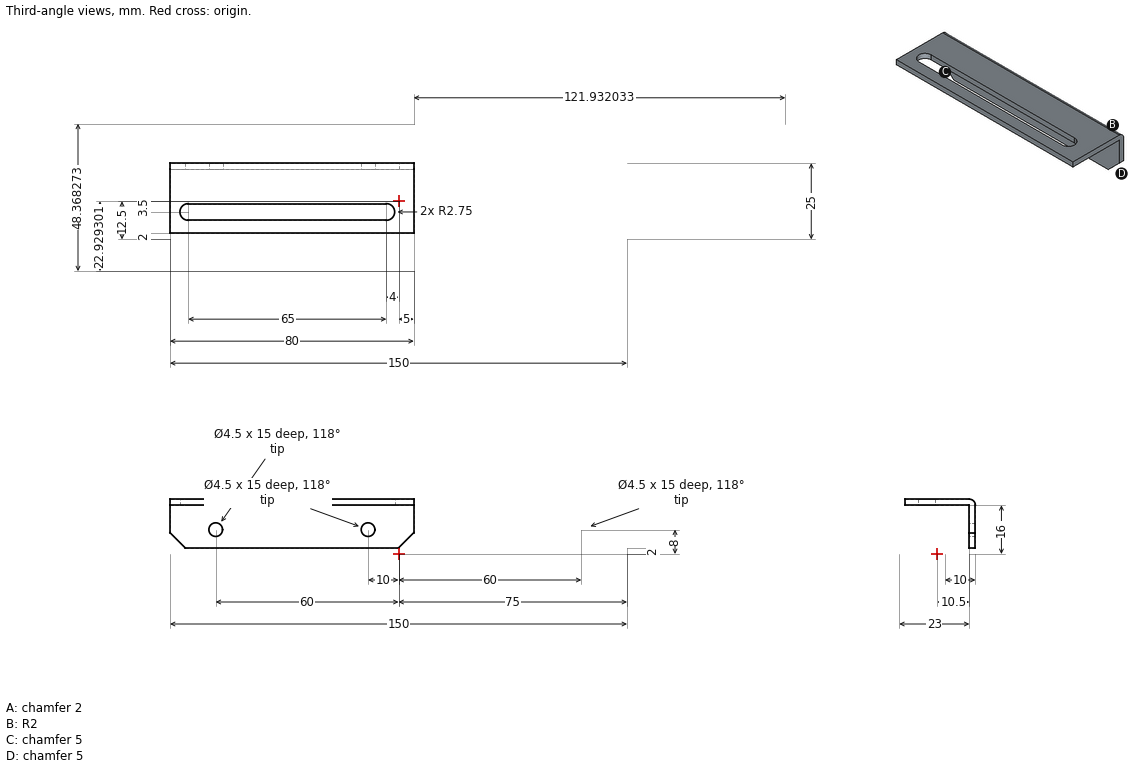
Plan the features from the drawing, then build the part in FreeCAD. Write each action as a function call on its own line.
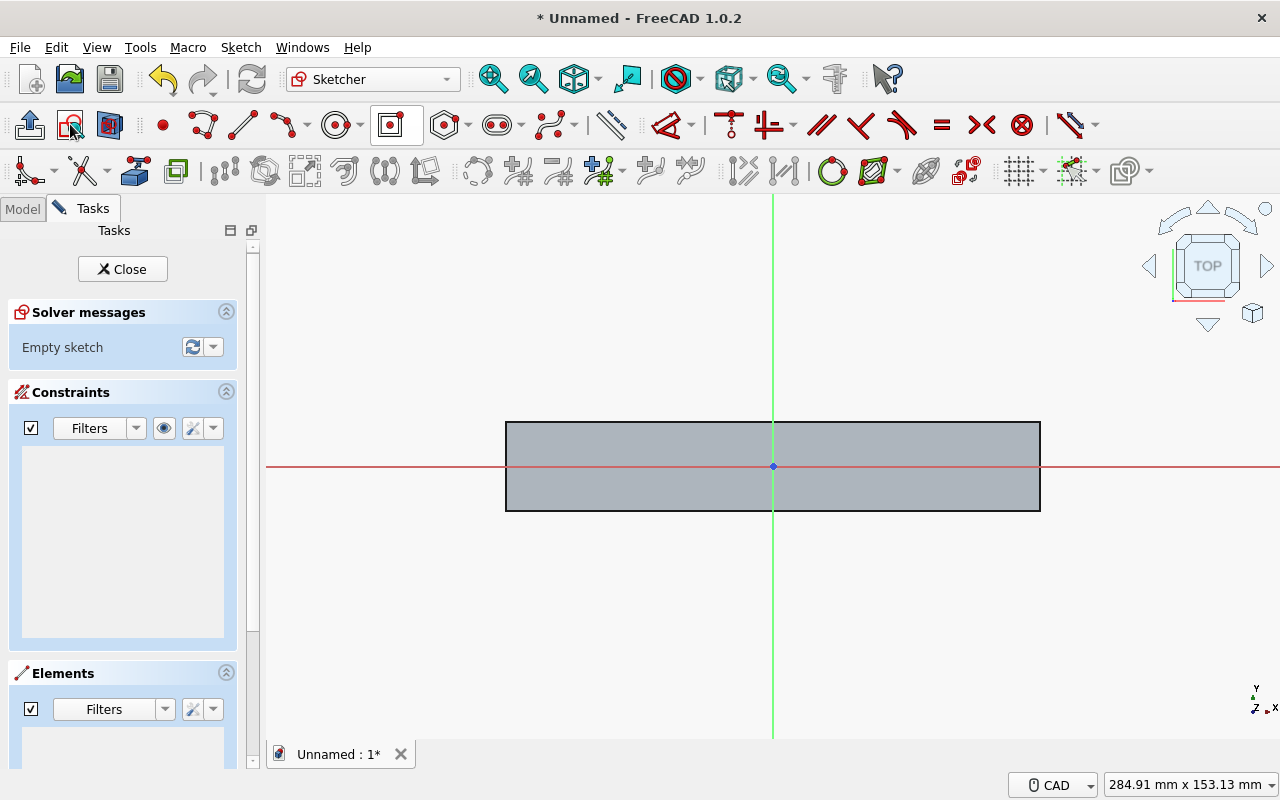
scroll(597, 487, up, 4)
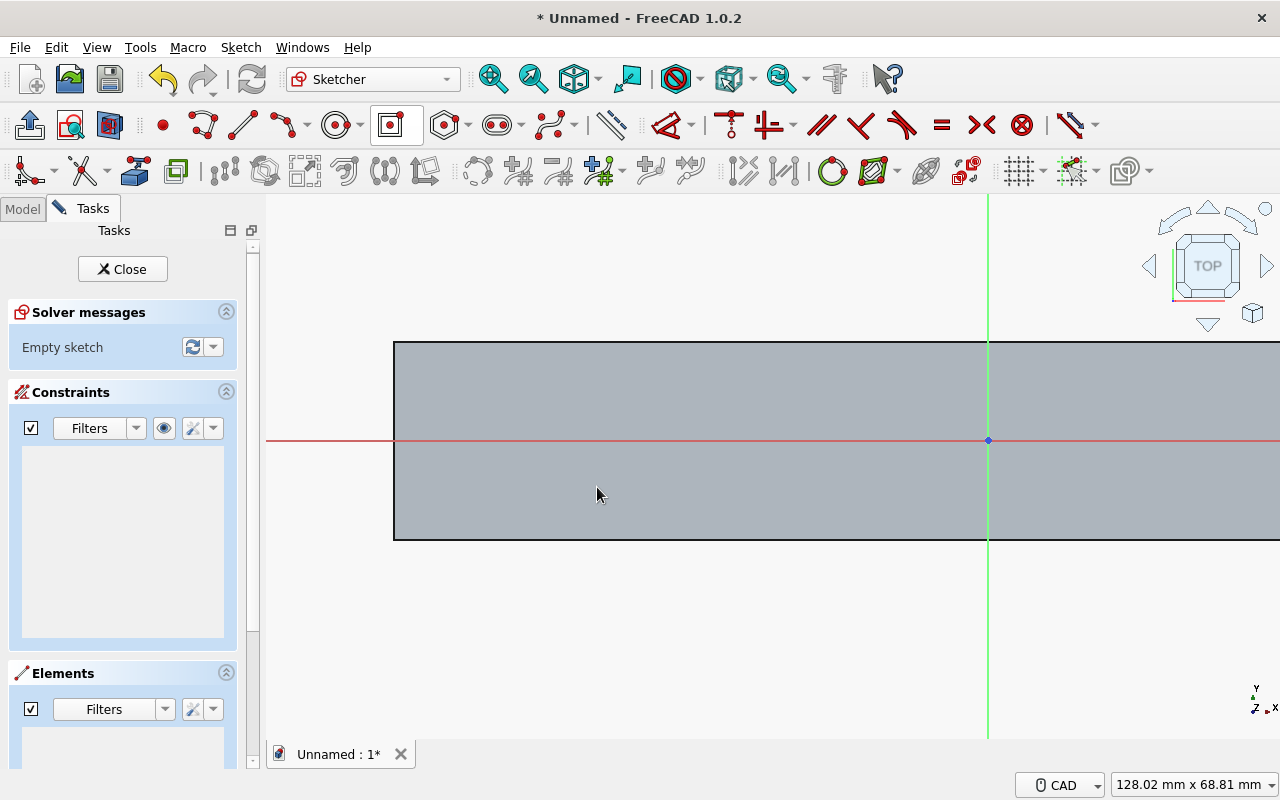
click(498, 126)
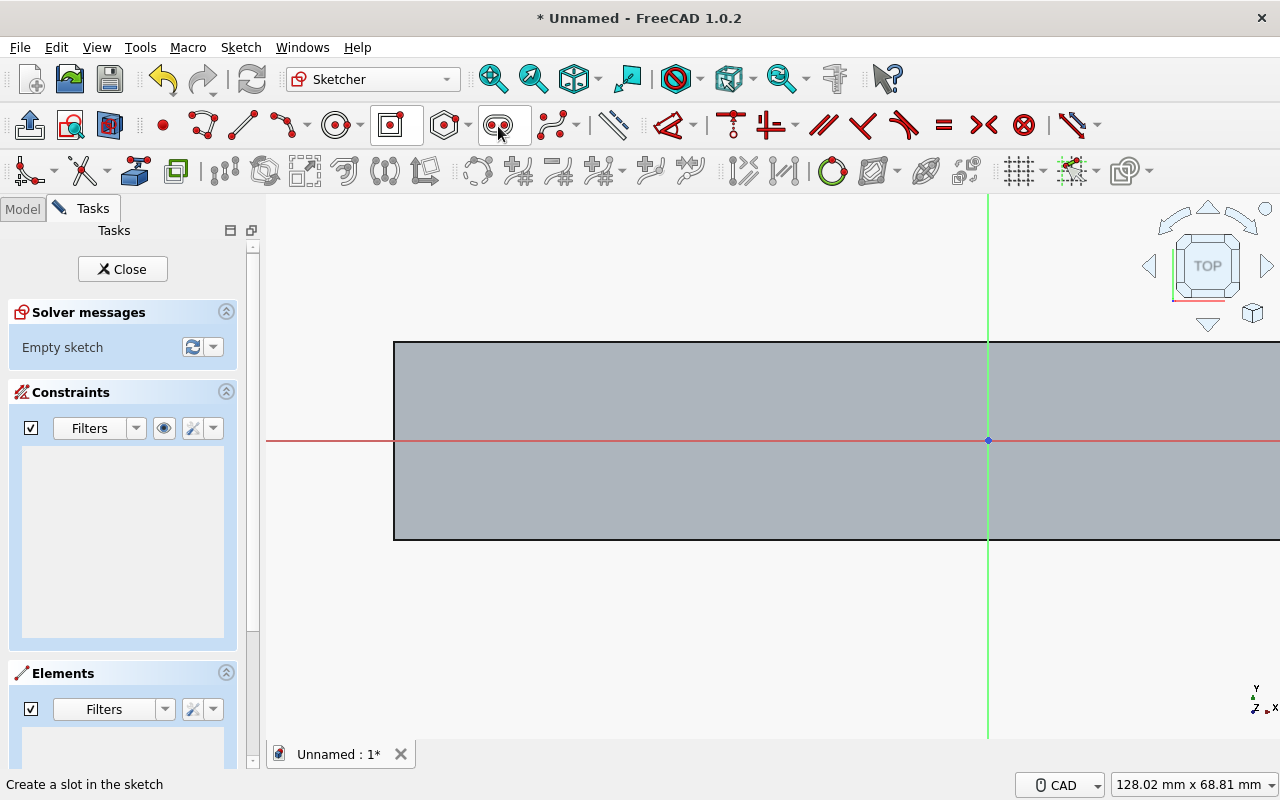
click(442, 468)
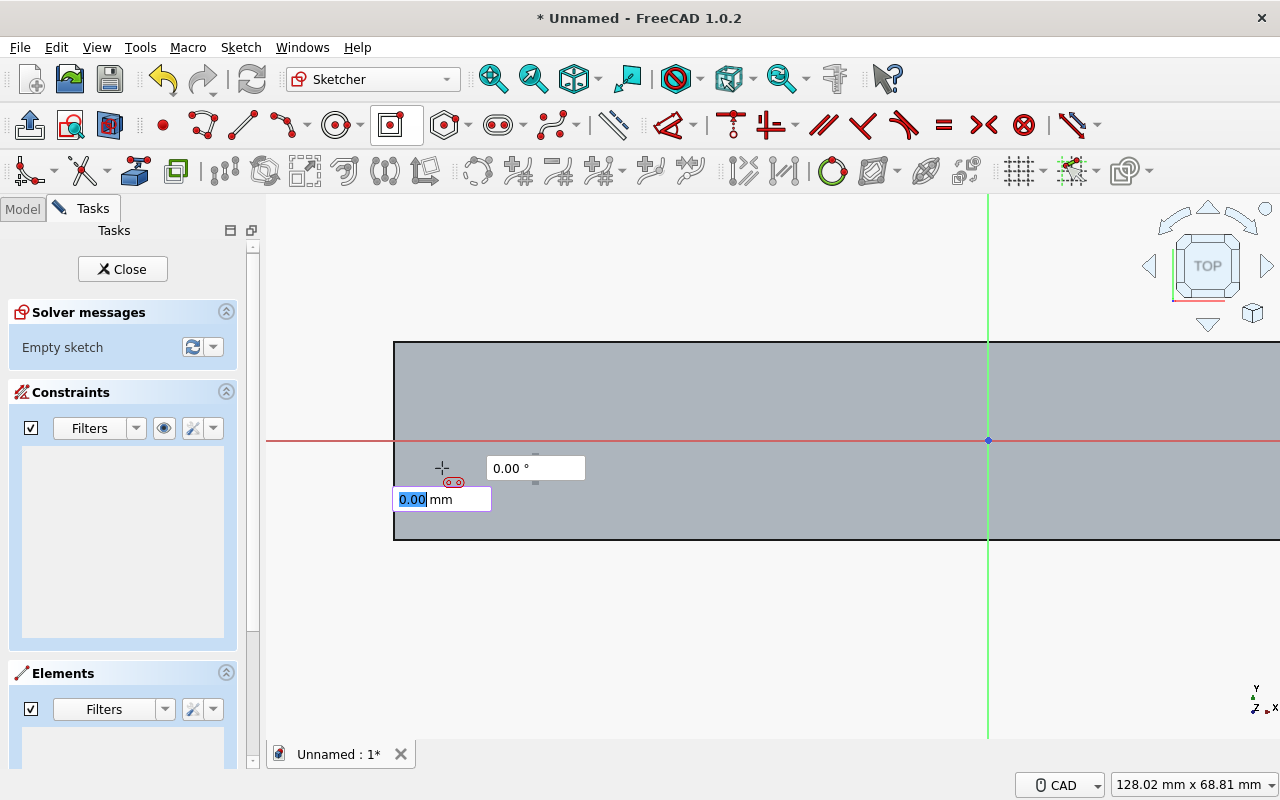
click(957, 468)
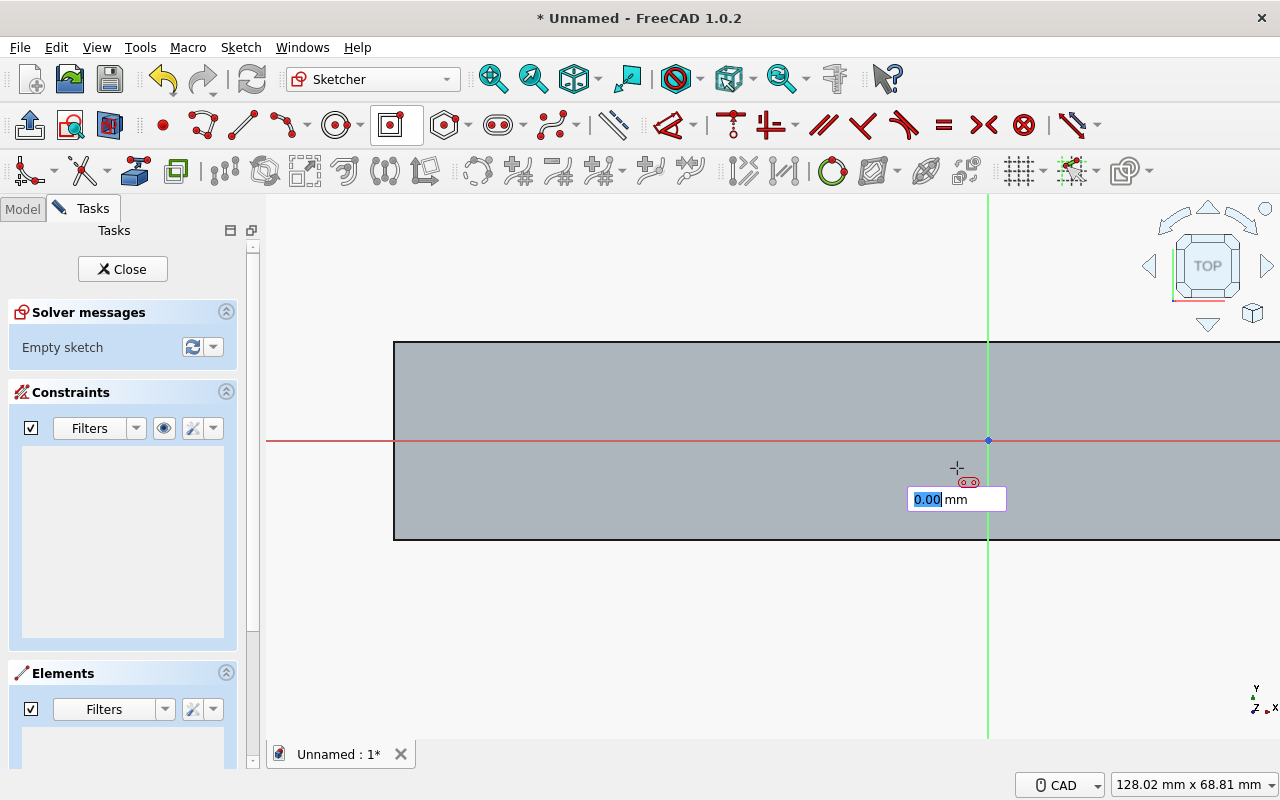
click(699, 490)
key(Escape)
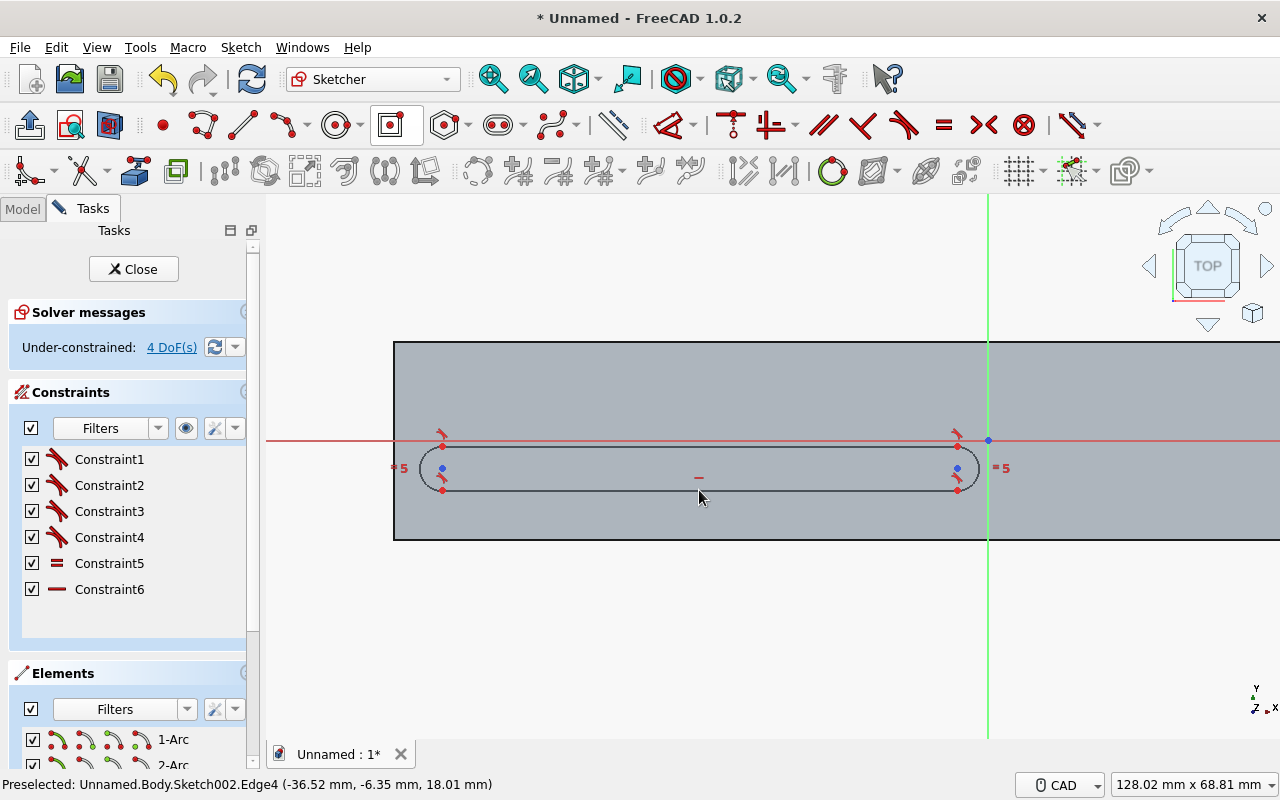
click(668, 126)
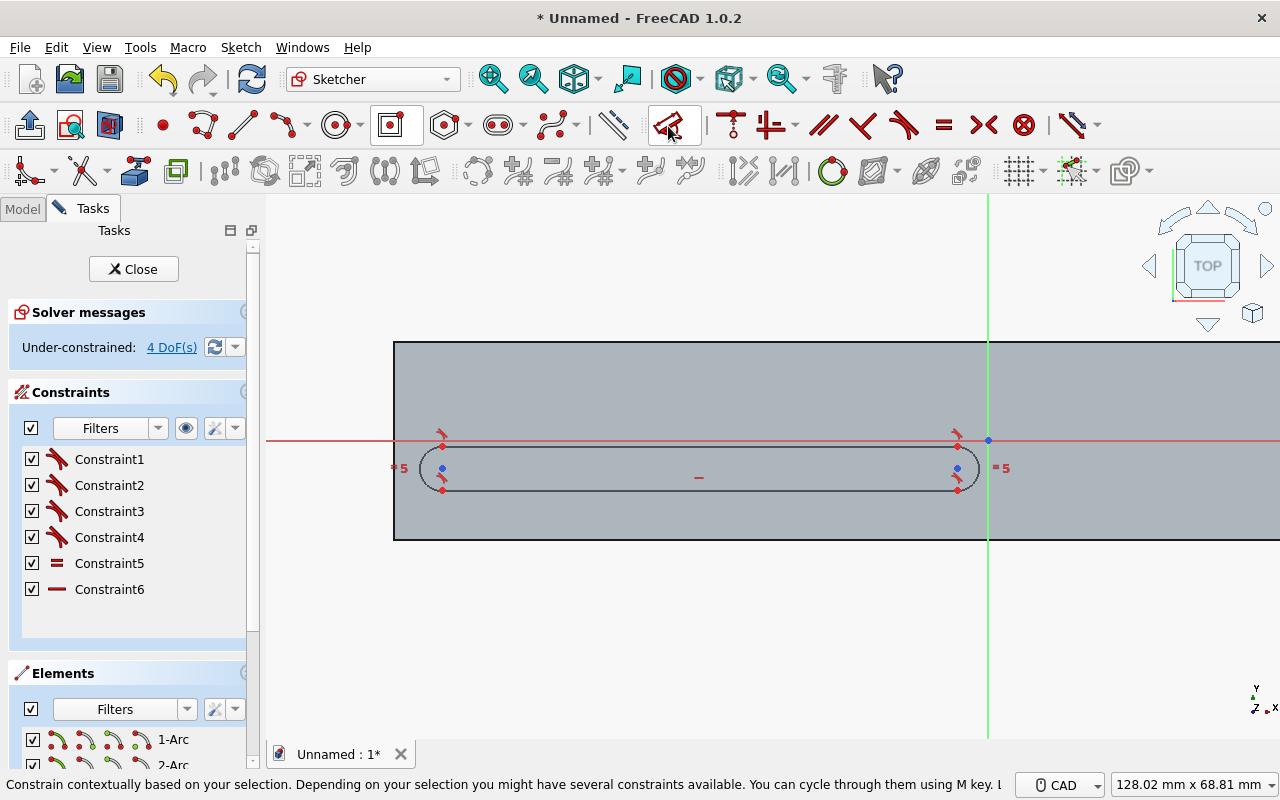
scroll(424, 456, up, 4)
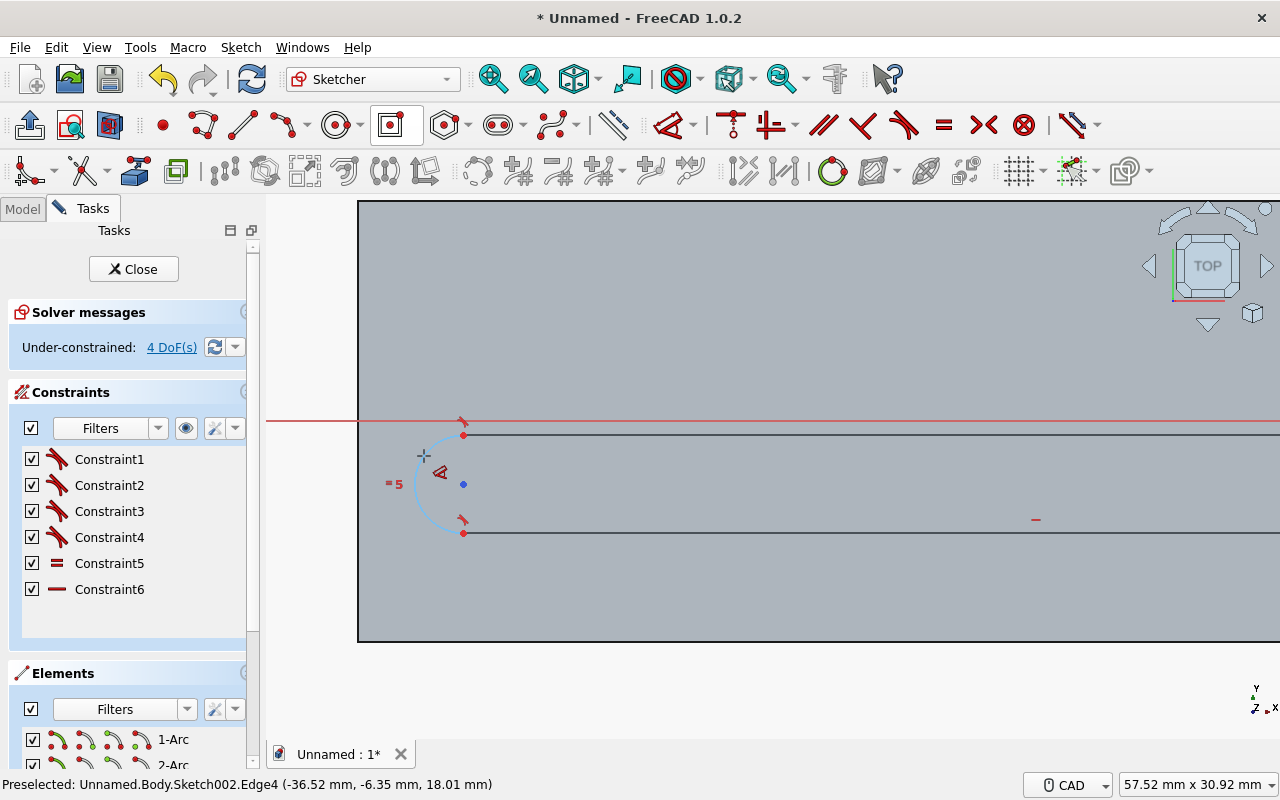
click(424, 456)
click(398, 437)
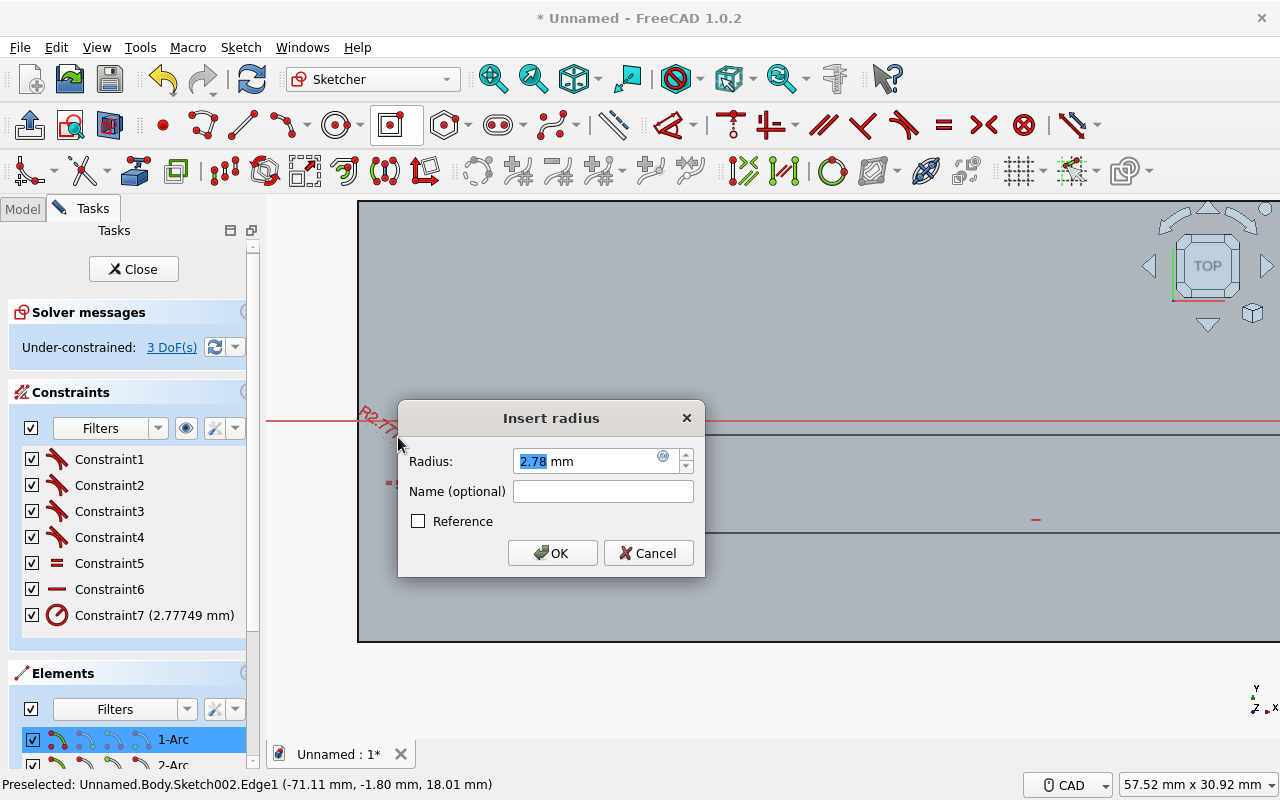
text(2.75)
key(Return)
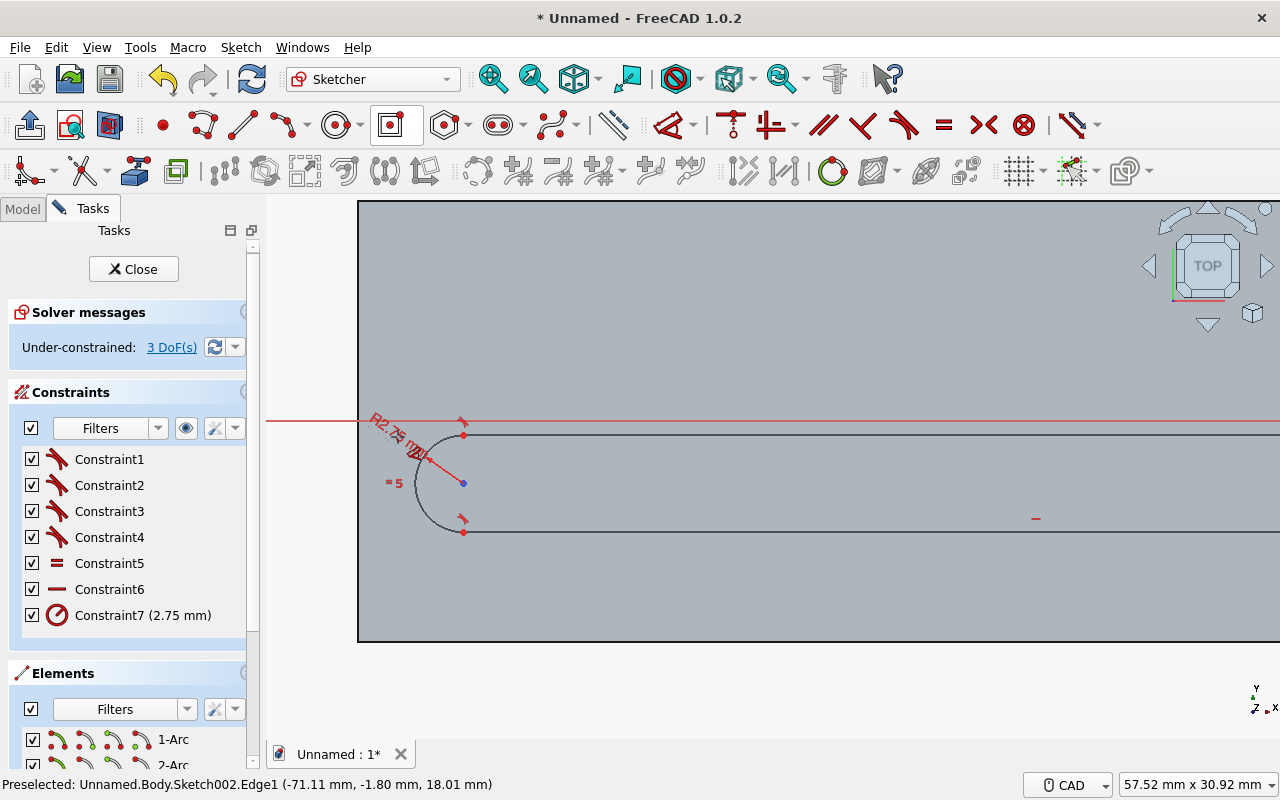
click(808, 435)
click(789, 401)